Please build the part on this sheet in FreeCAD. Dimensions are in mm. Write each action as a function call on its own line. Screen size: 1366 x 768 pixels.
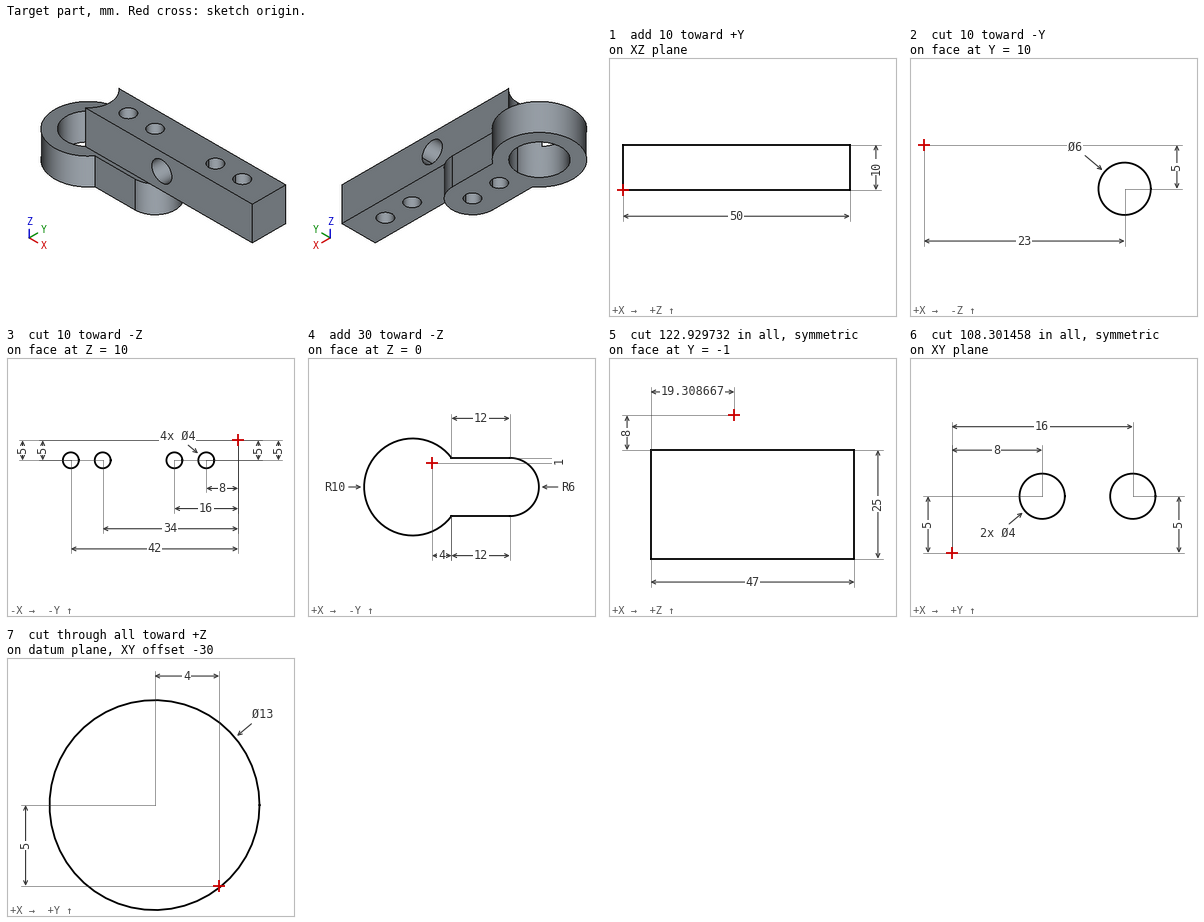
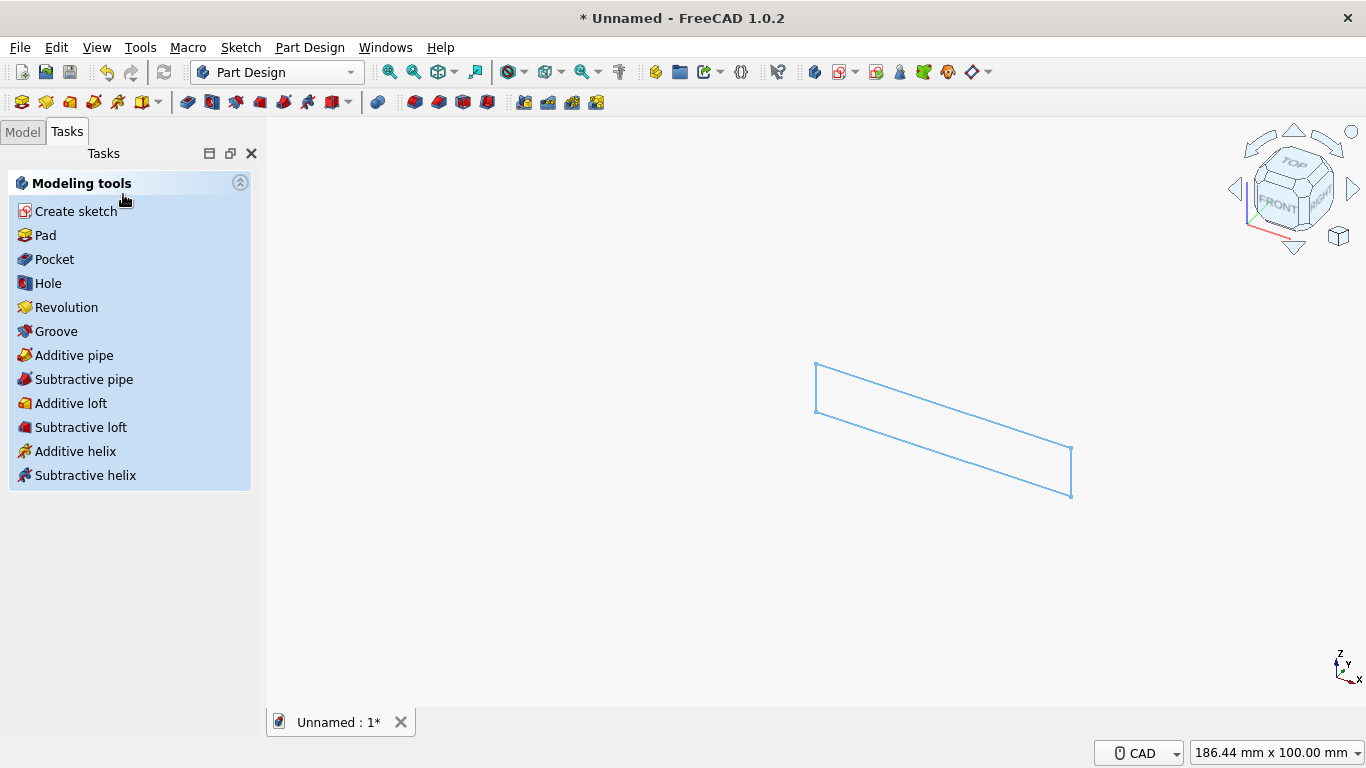
click(22, 102)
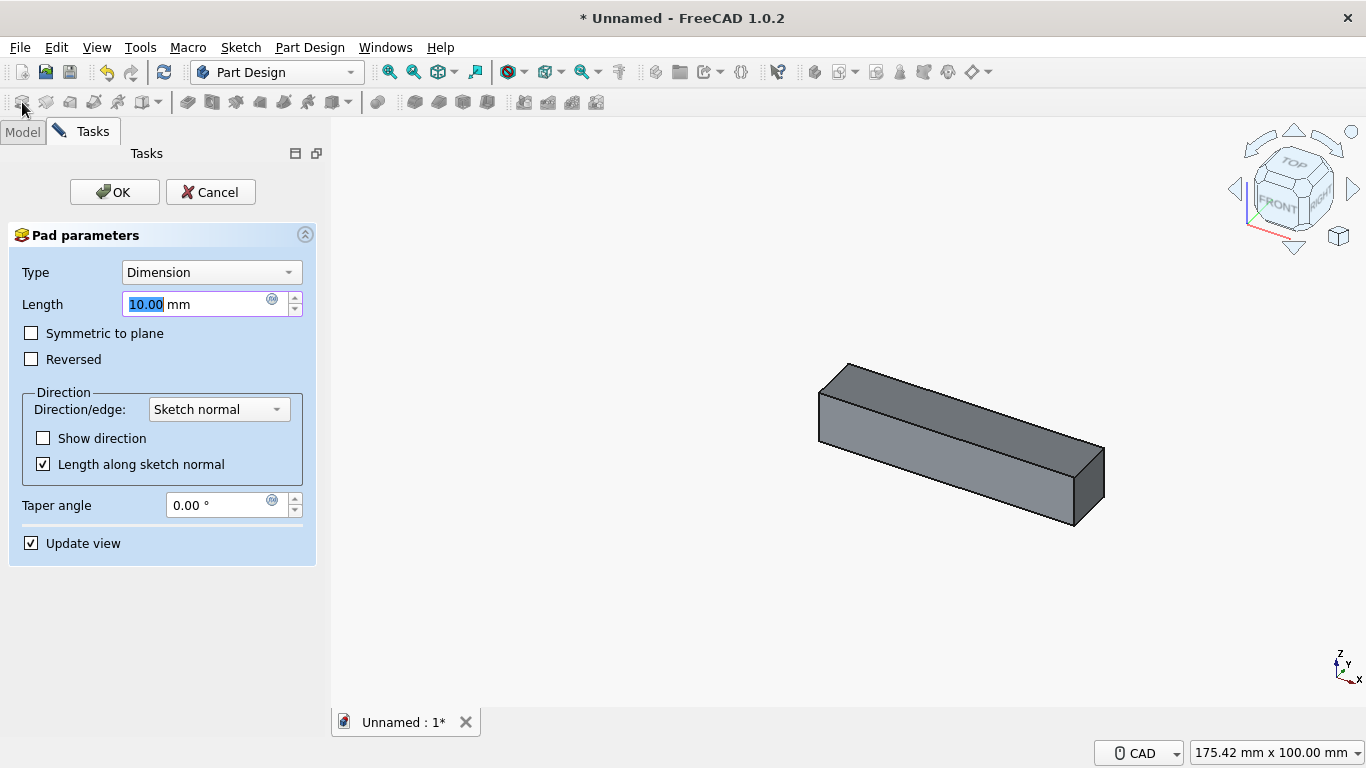
text(10)
key(Tab)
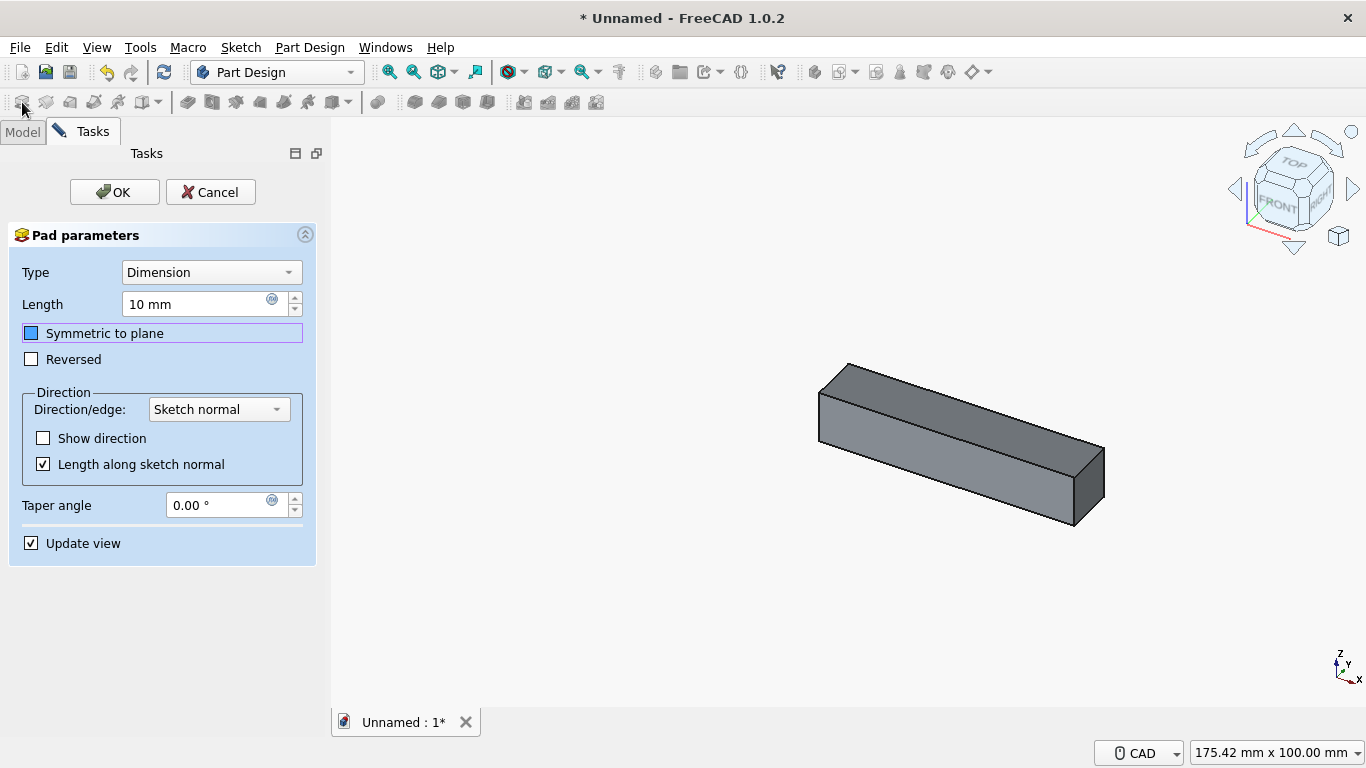
click(30, 359)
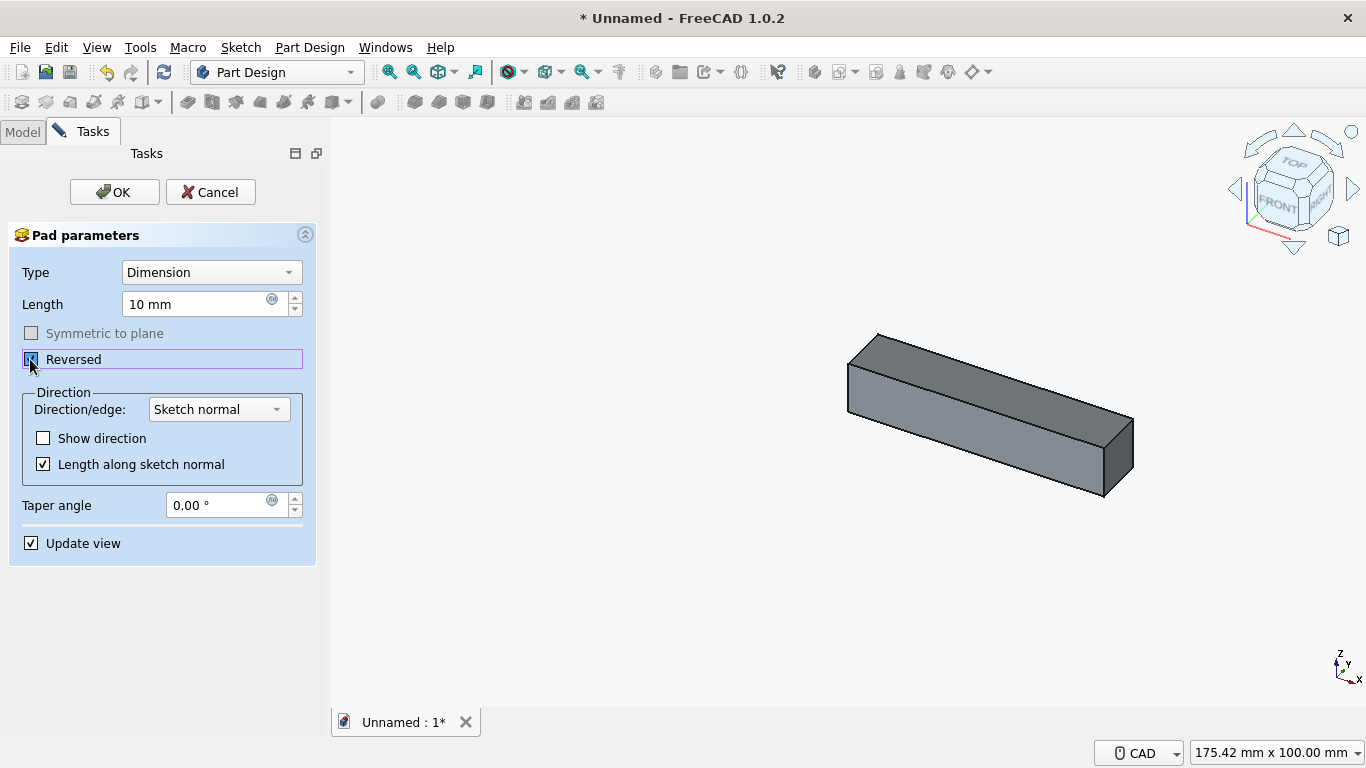
click(115, 192)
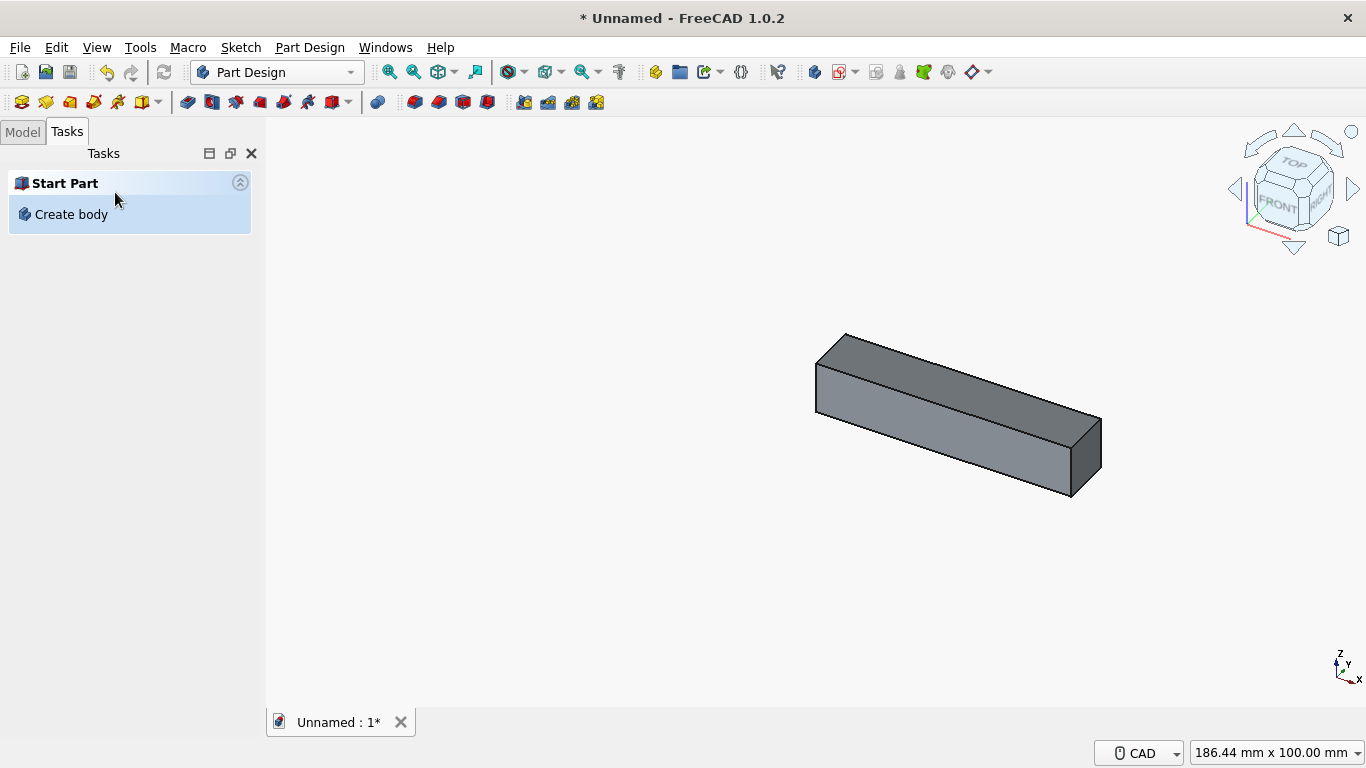
click(390, 72)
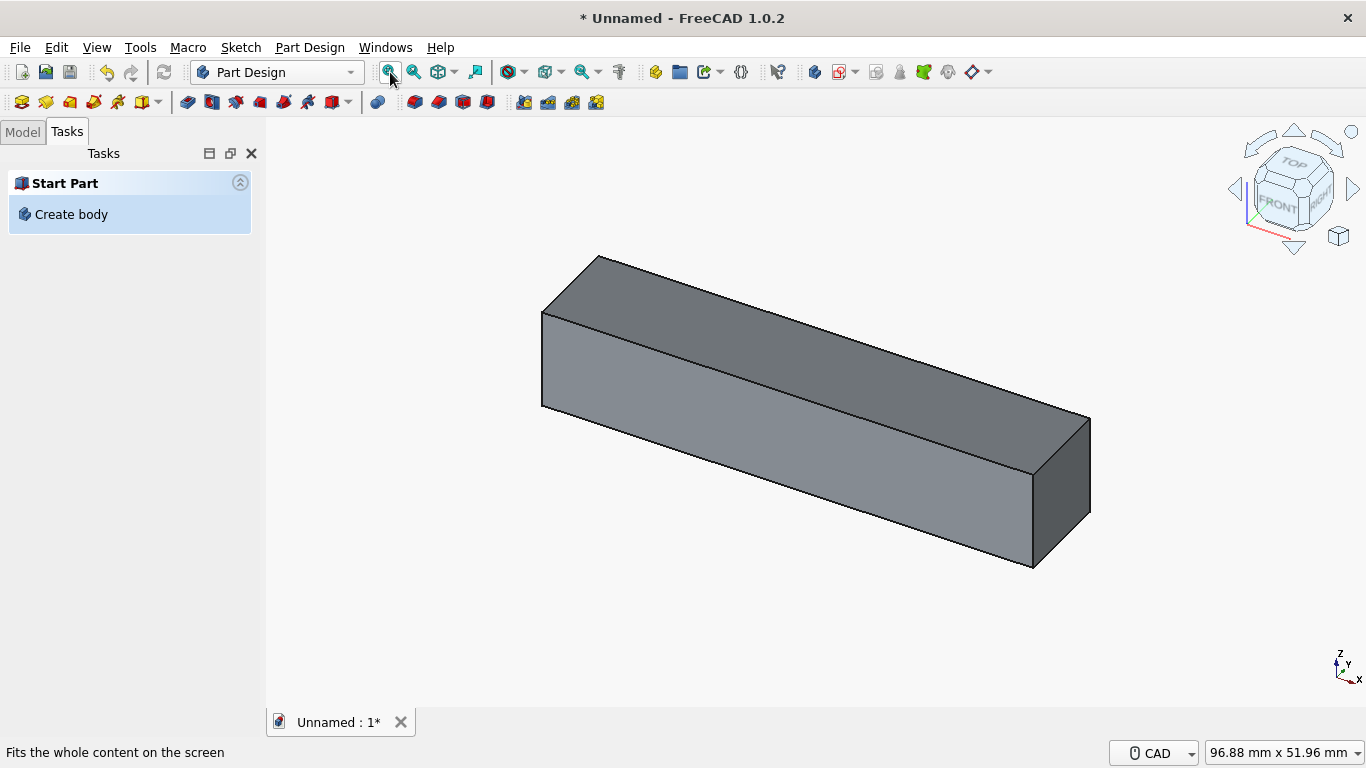
key(4)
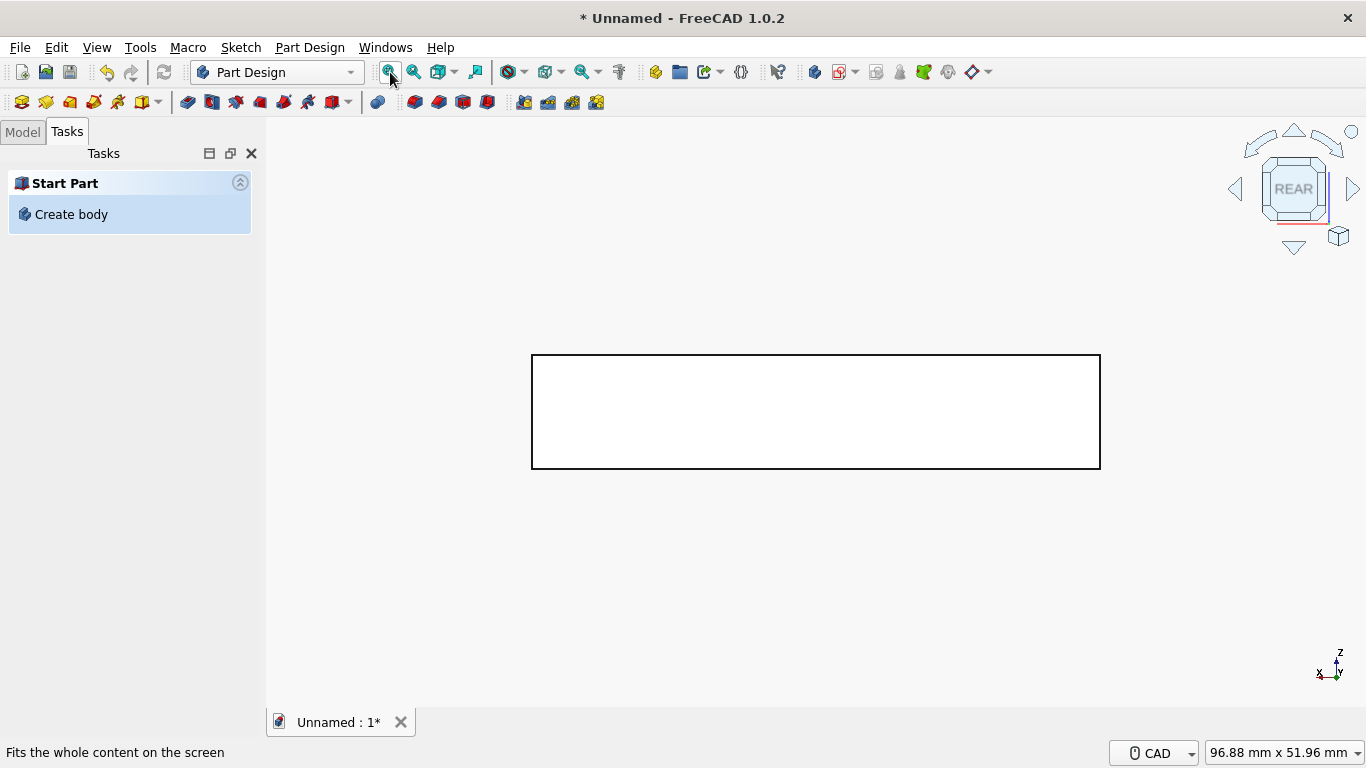
click(654, 411)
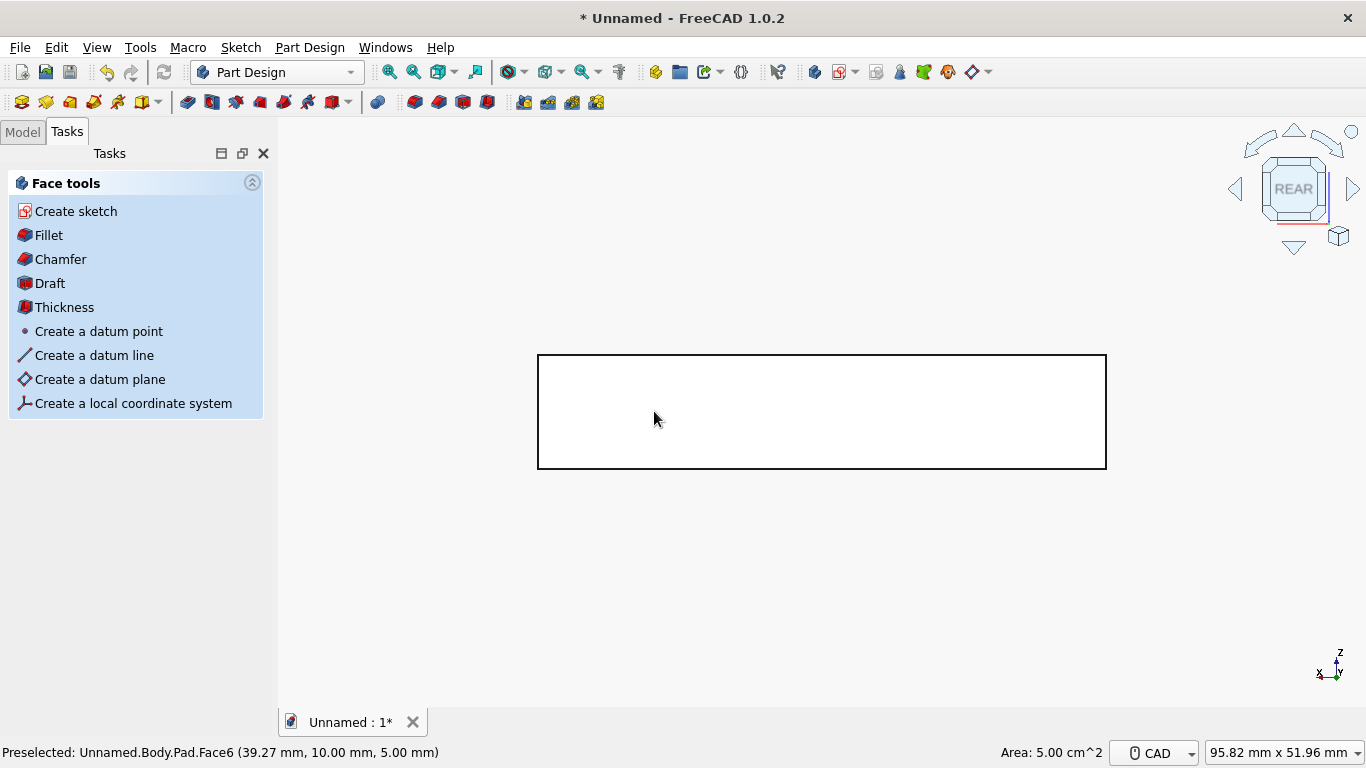
click(840, 72)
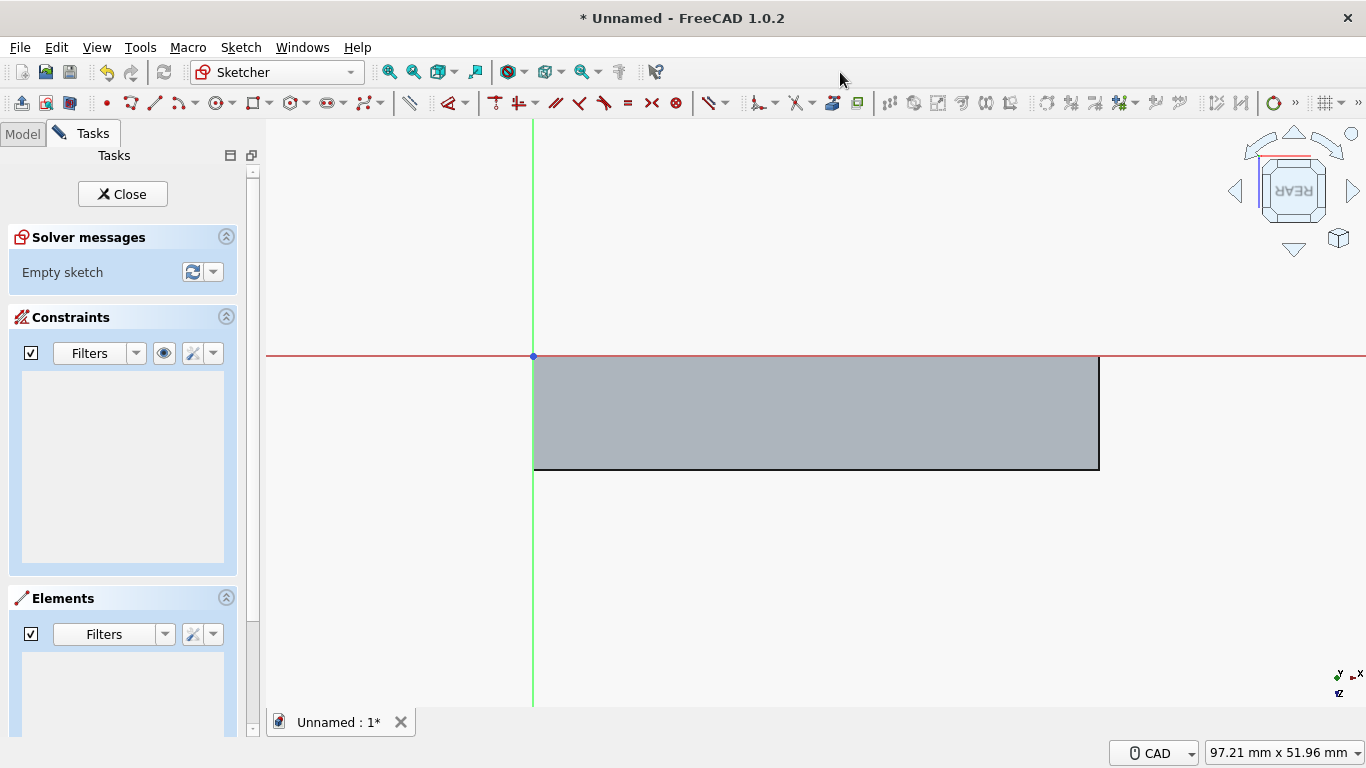
scroll(802, 413, up, 9)